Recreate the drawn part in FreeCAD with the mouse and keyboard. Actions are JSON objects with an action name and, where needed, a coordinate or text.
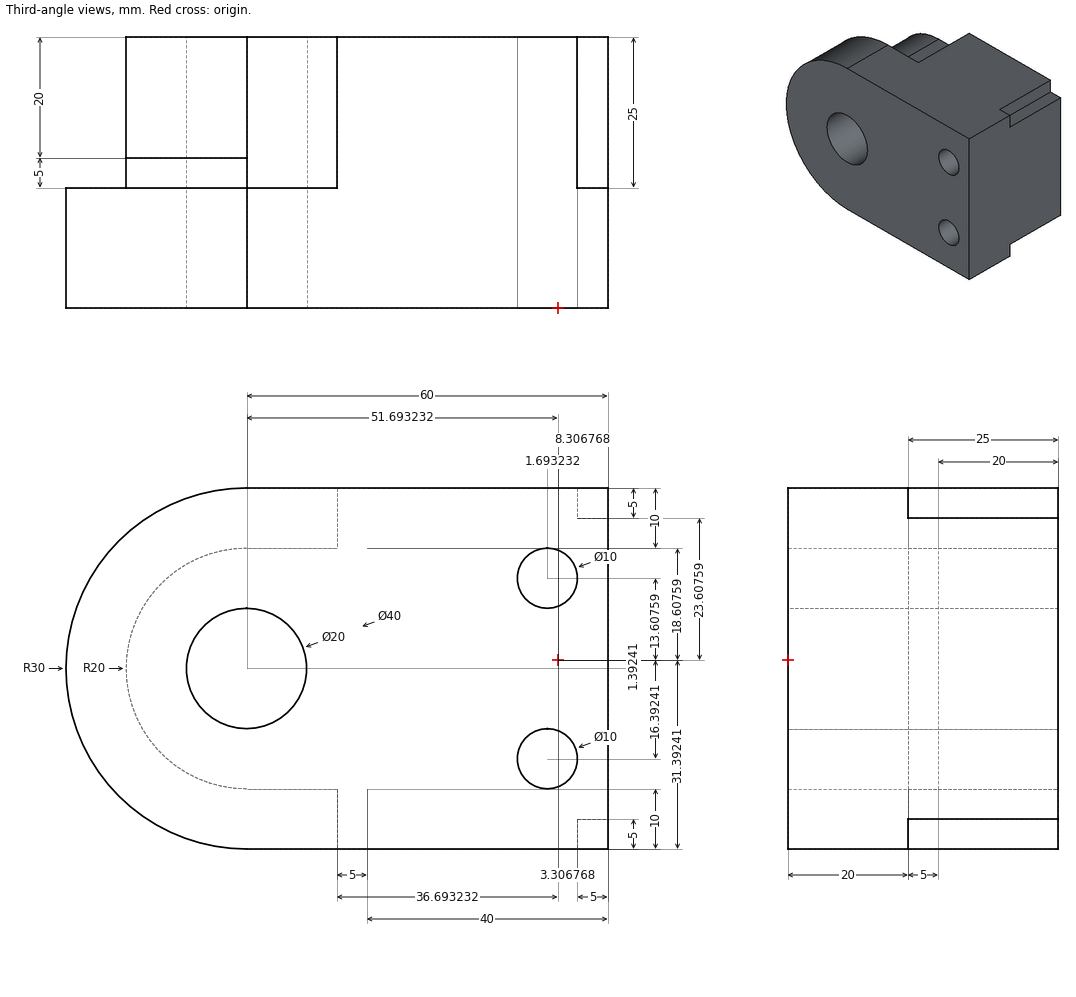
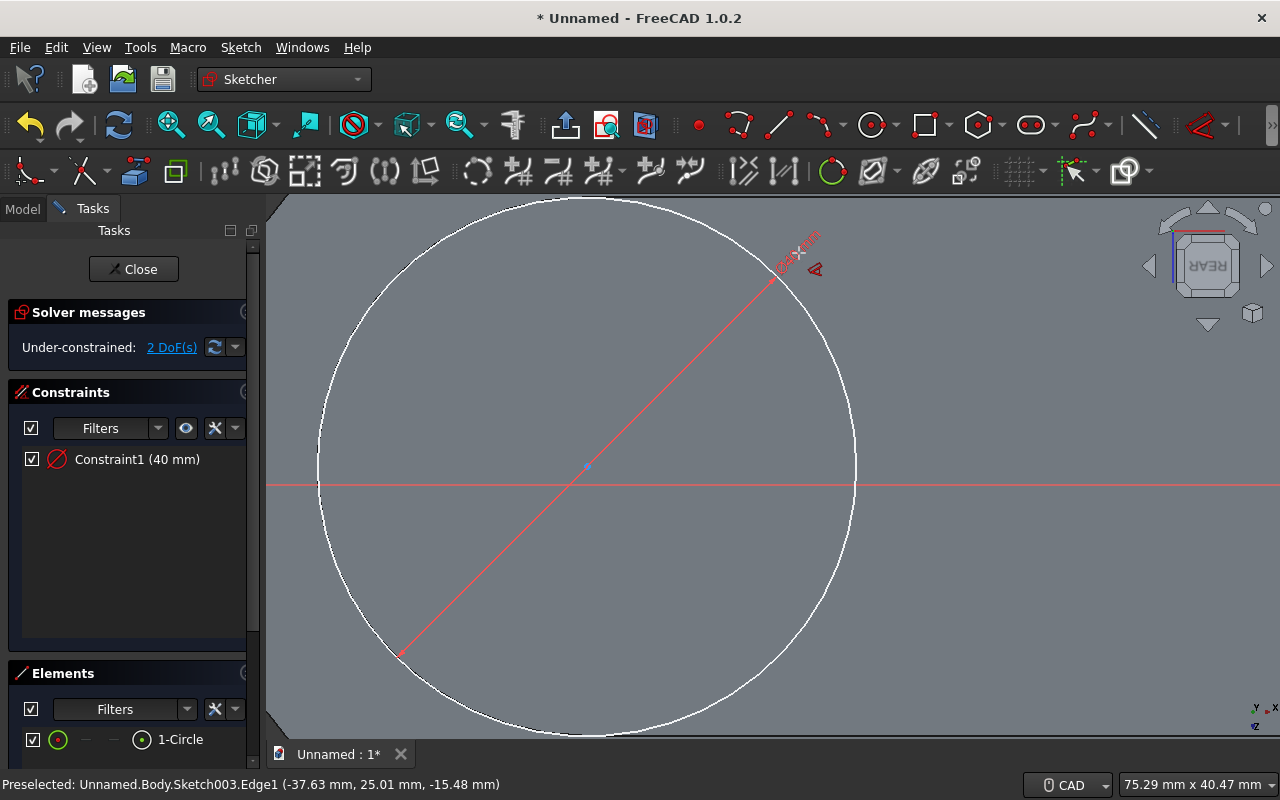
{"action": "scroll", "coordinate": [587, 467], "scroll_direction": "up", "scroll_amount": 4}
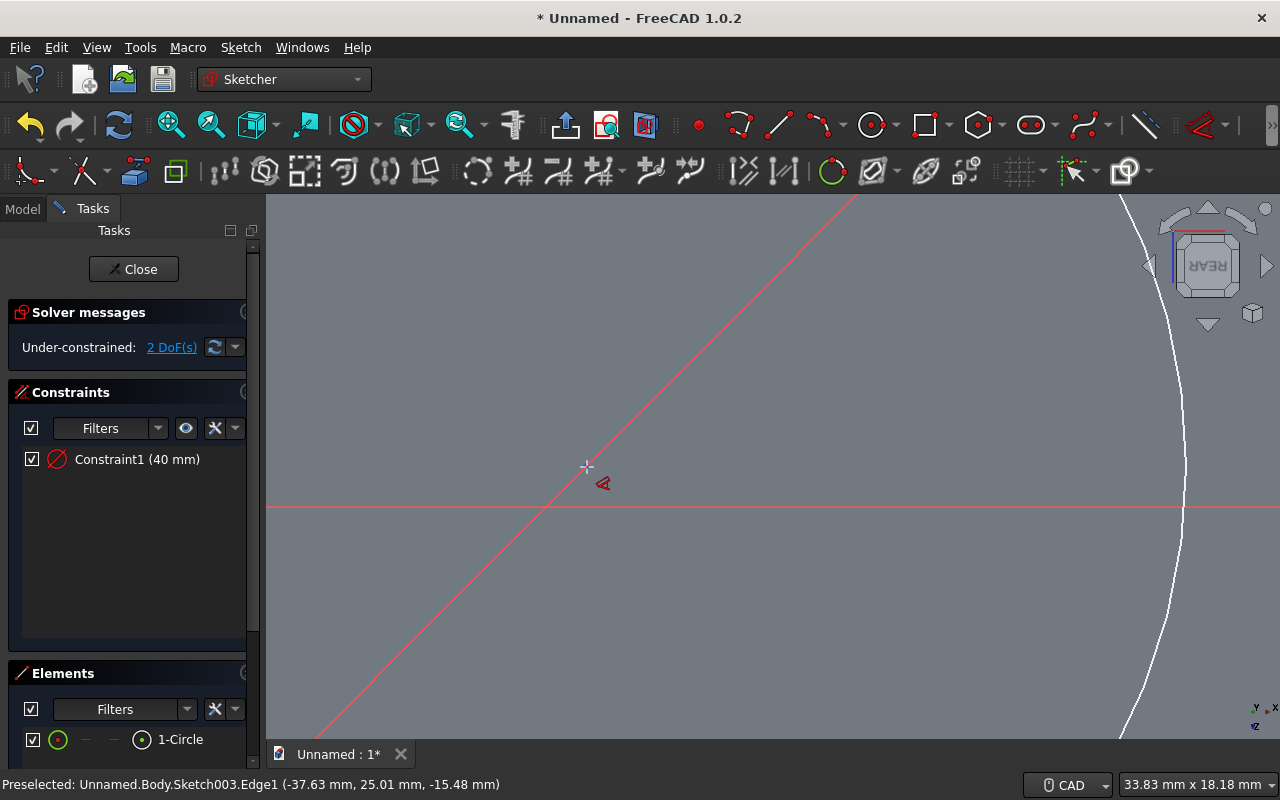
{"action": "left_click", "coordinate": [587, 466]}
{"action": "left_click", "coordinate": [553, 487]}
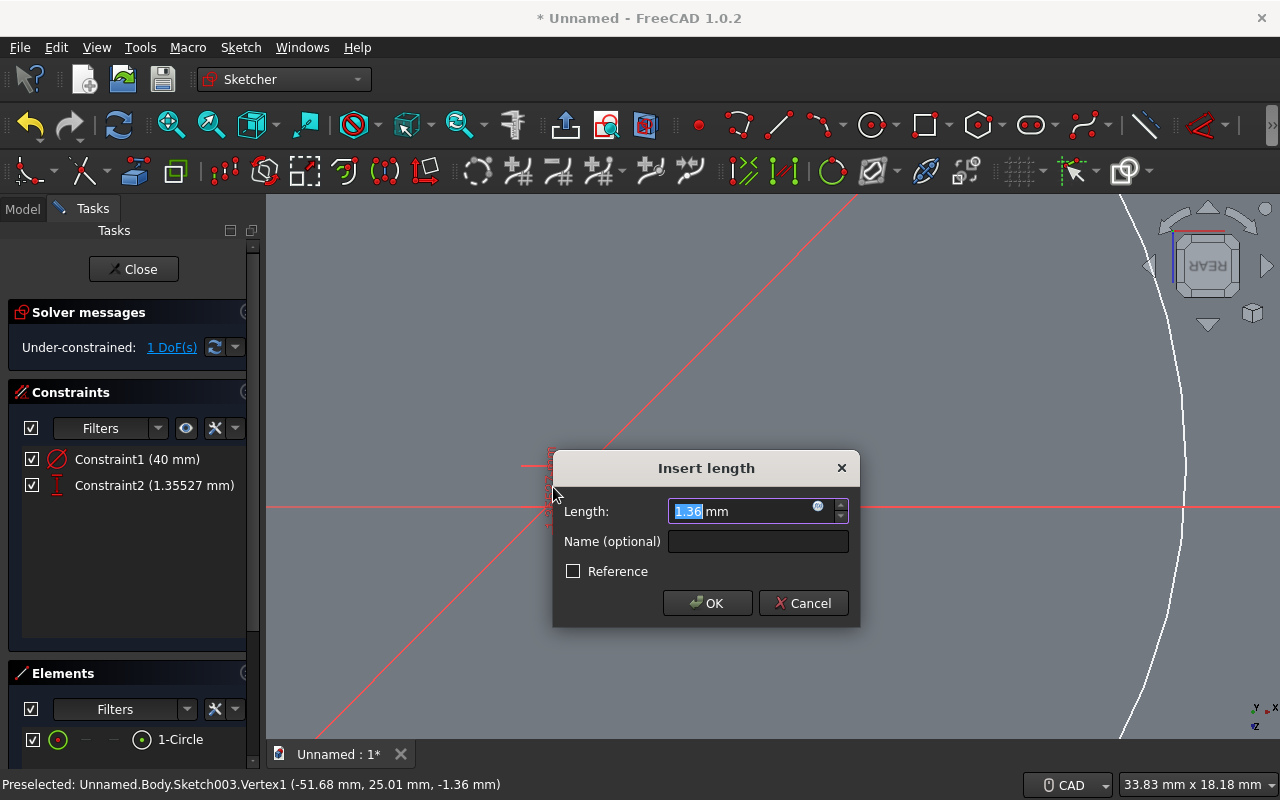
{"action": "type", "text": "1.39241"}
{"action": "key", "text": "Return"}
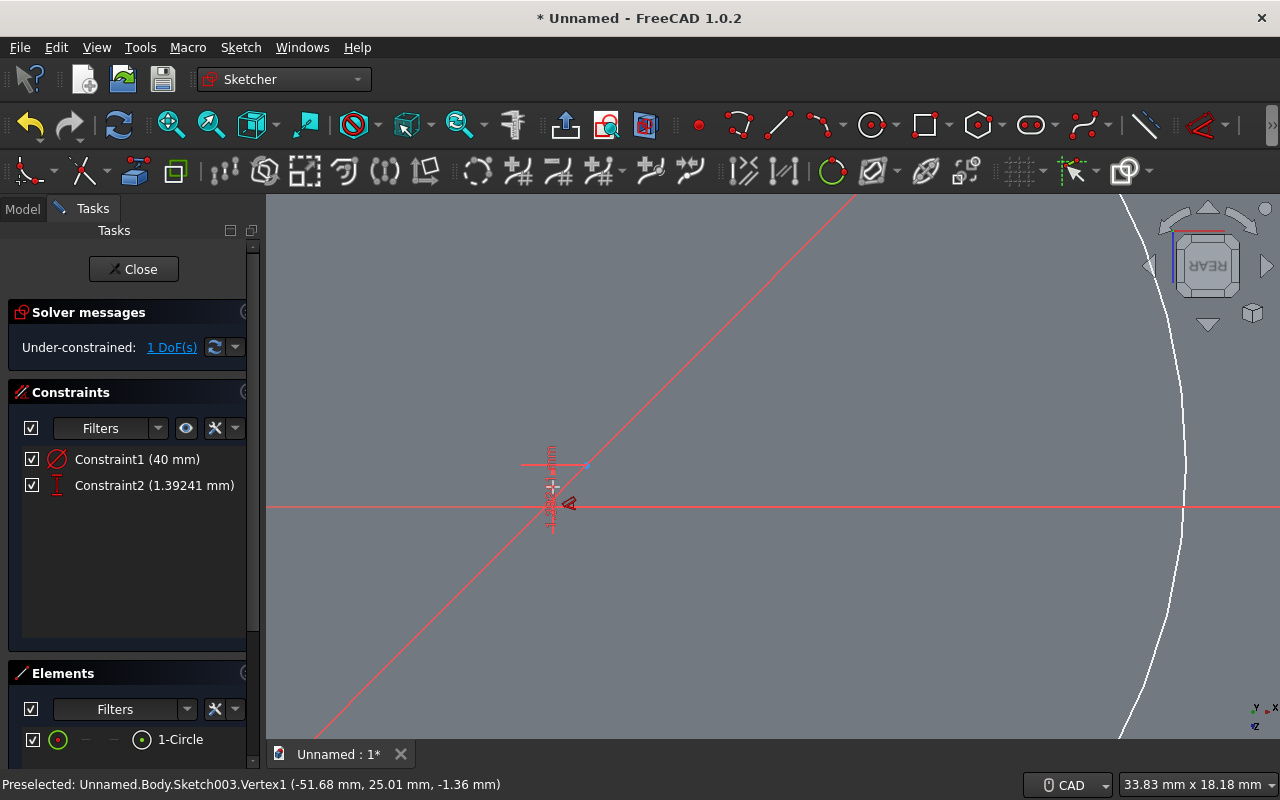
{"action": "scroll", "coordinate": [588, 467], "scroll_direction": "down", "scroll_amount": 7}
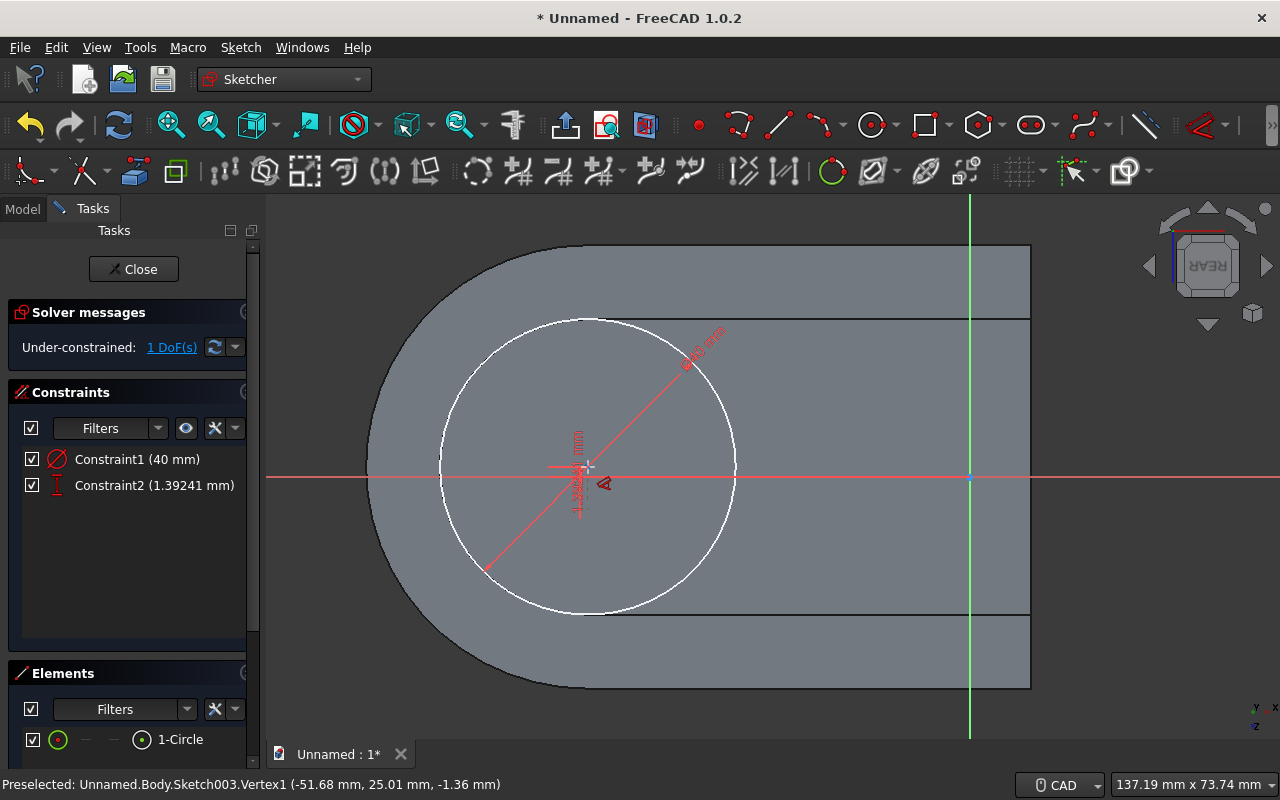
{"action": "left_click", "coordinate": [588, 467]}
{"action": "left_click", "coordinate": [779, 511]}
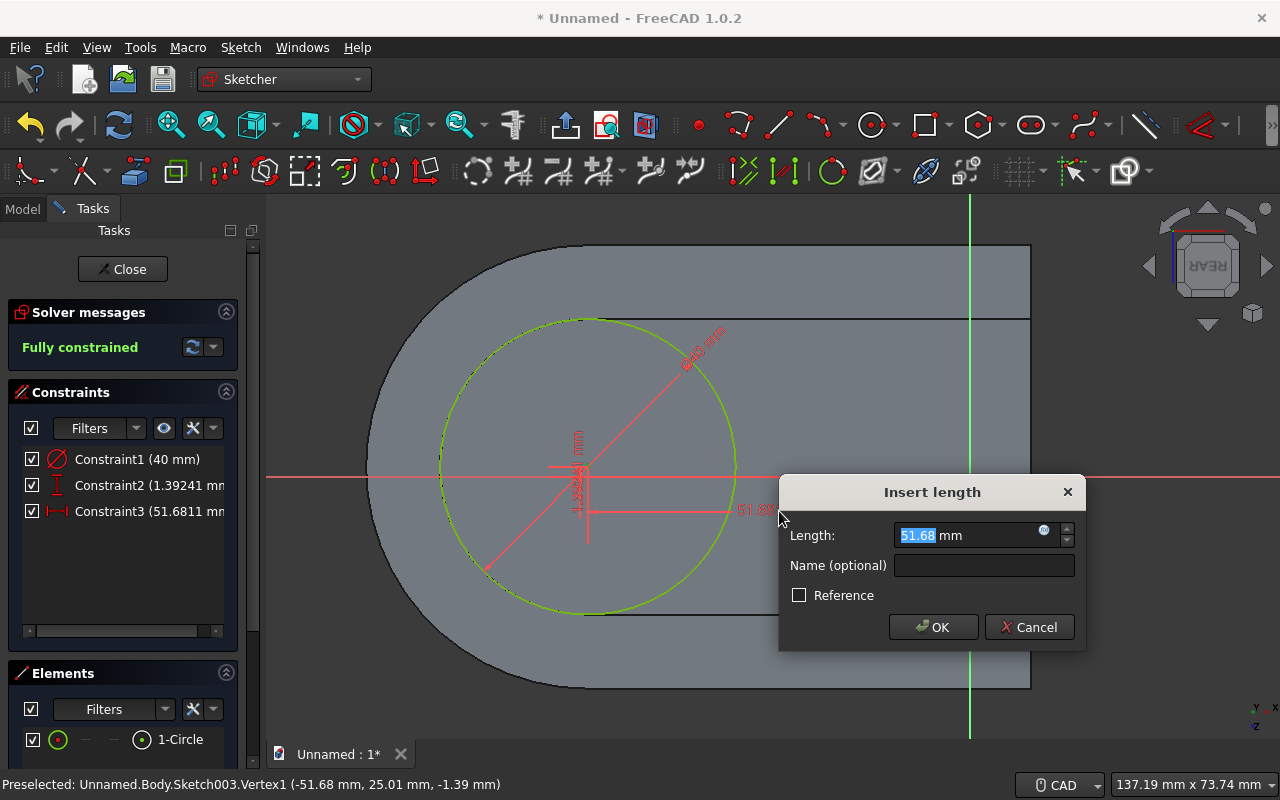
{"action": "type", "text": "51.693232"}
{"action": "key", "text": "Return"}
{"action": "key", "text": "Escape"}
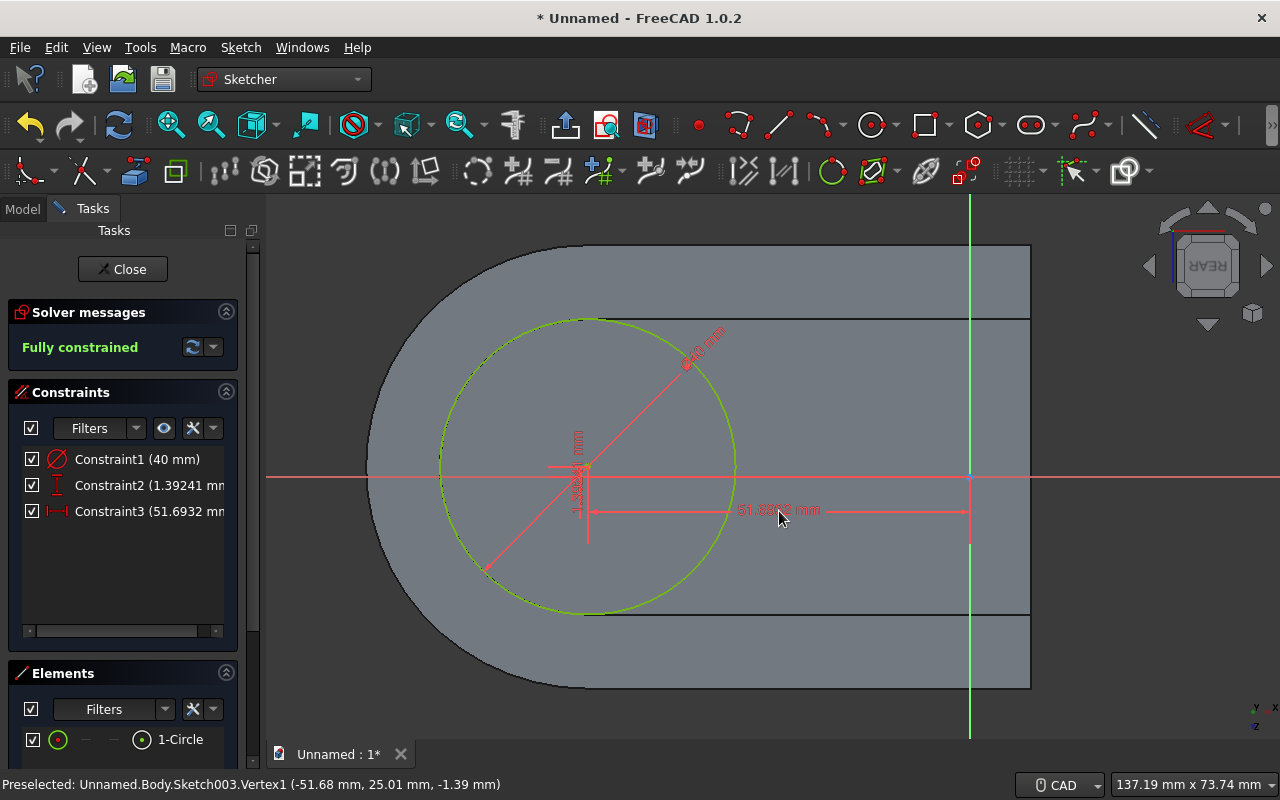
{"action": "left_click", "coordinate": [123, 269]}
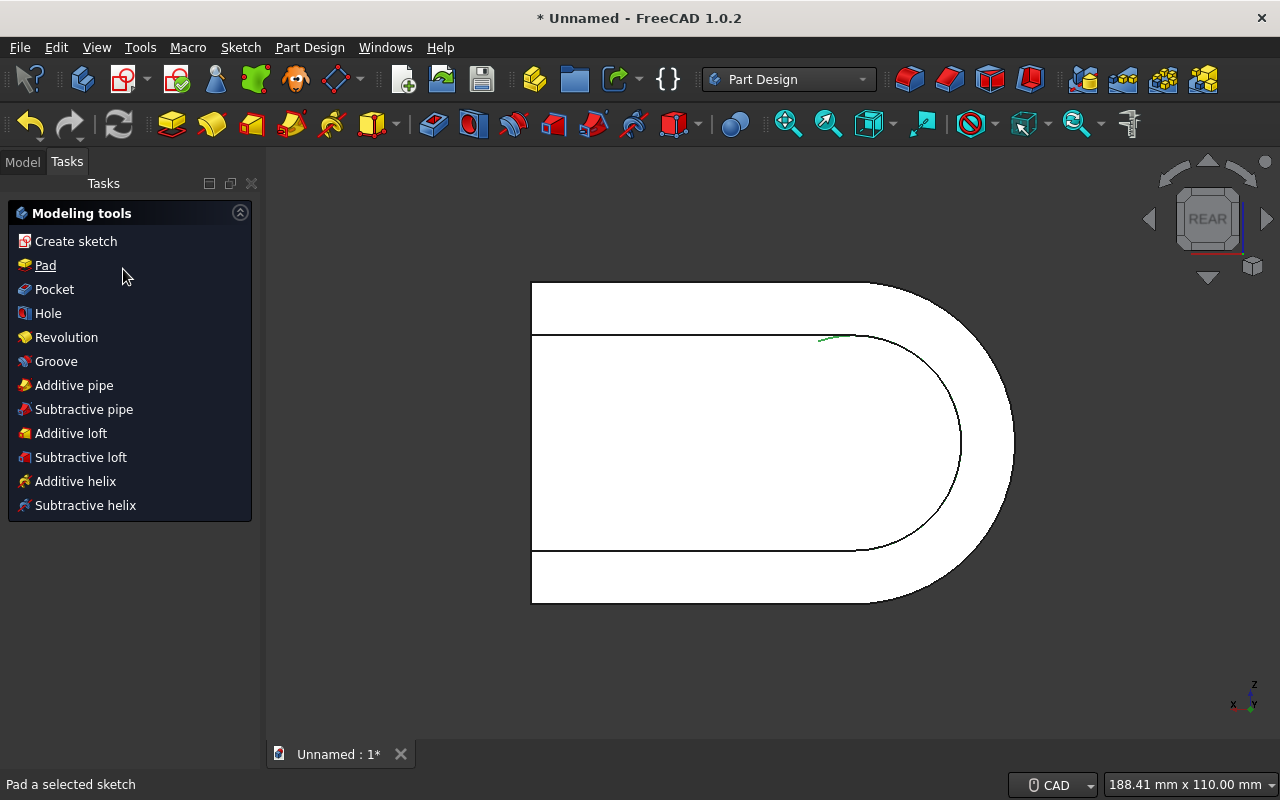
{"action": "left_click", "coordinate": [172, 124]}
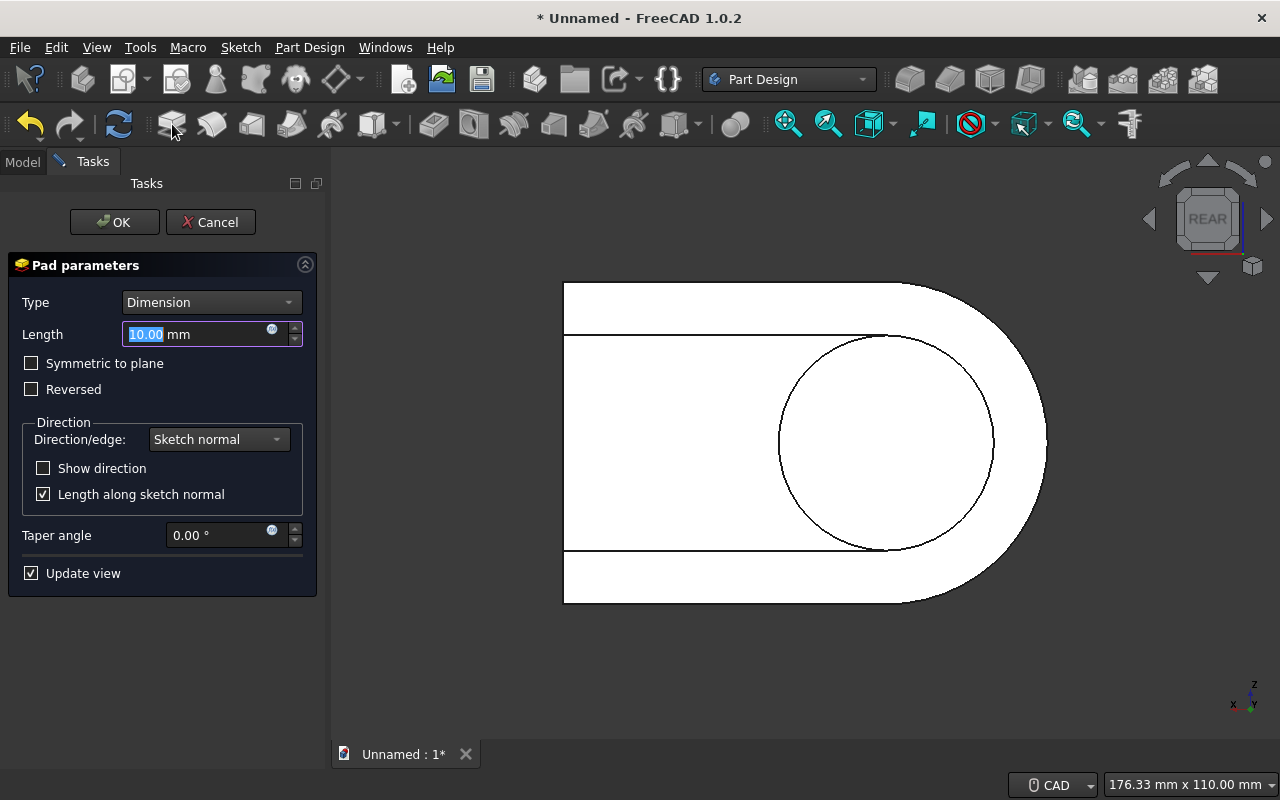
{"action": "type", "text": "20"}
{"action": "key", "text": "Tab"}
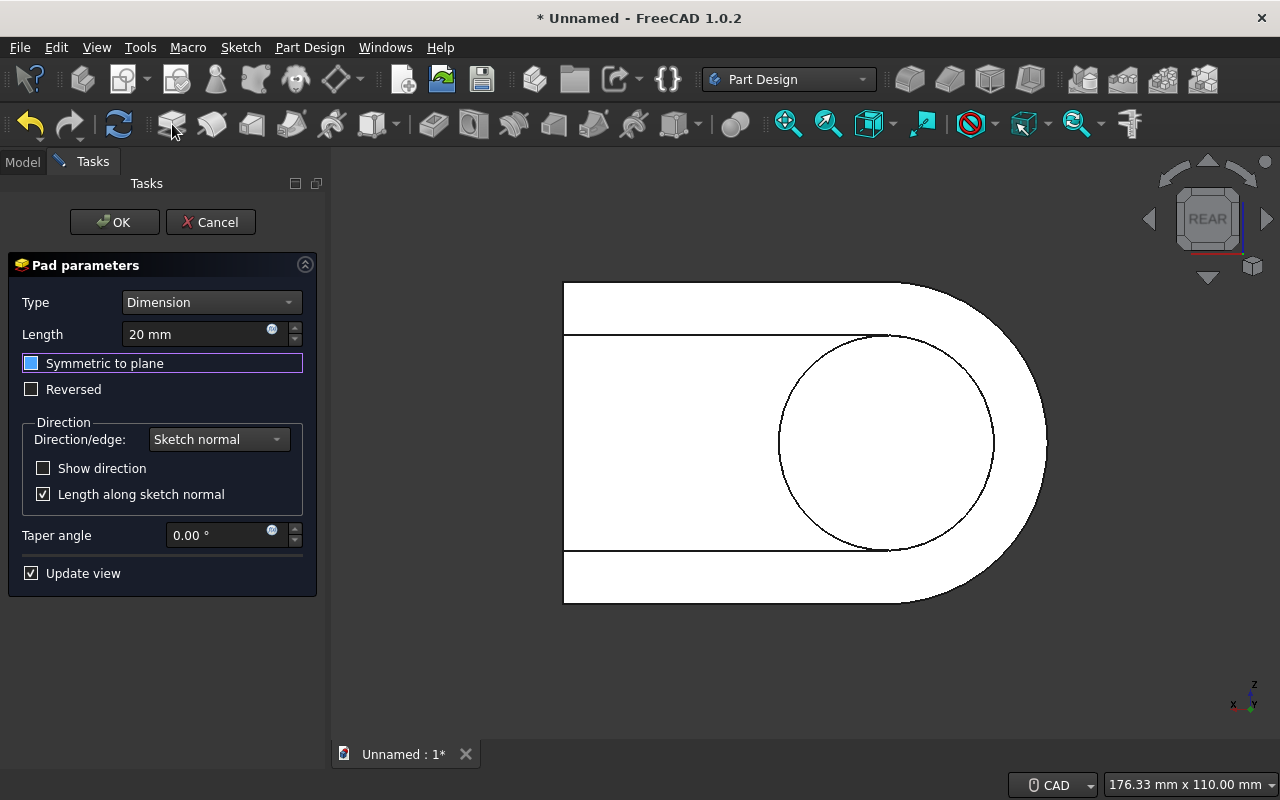
{"action": "left_click", "coordinate": [115, 222]}